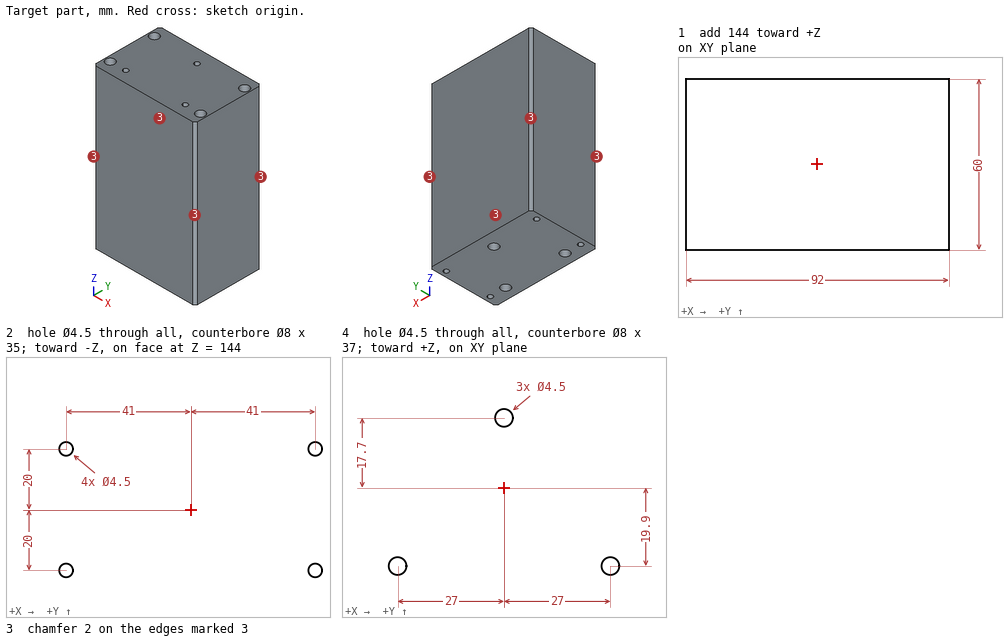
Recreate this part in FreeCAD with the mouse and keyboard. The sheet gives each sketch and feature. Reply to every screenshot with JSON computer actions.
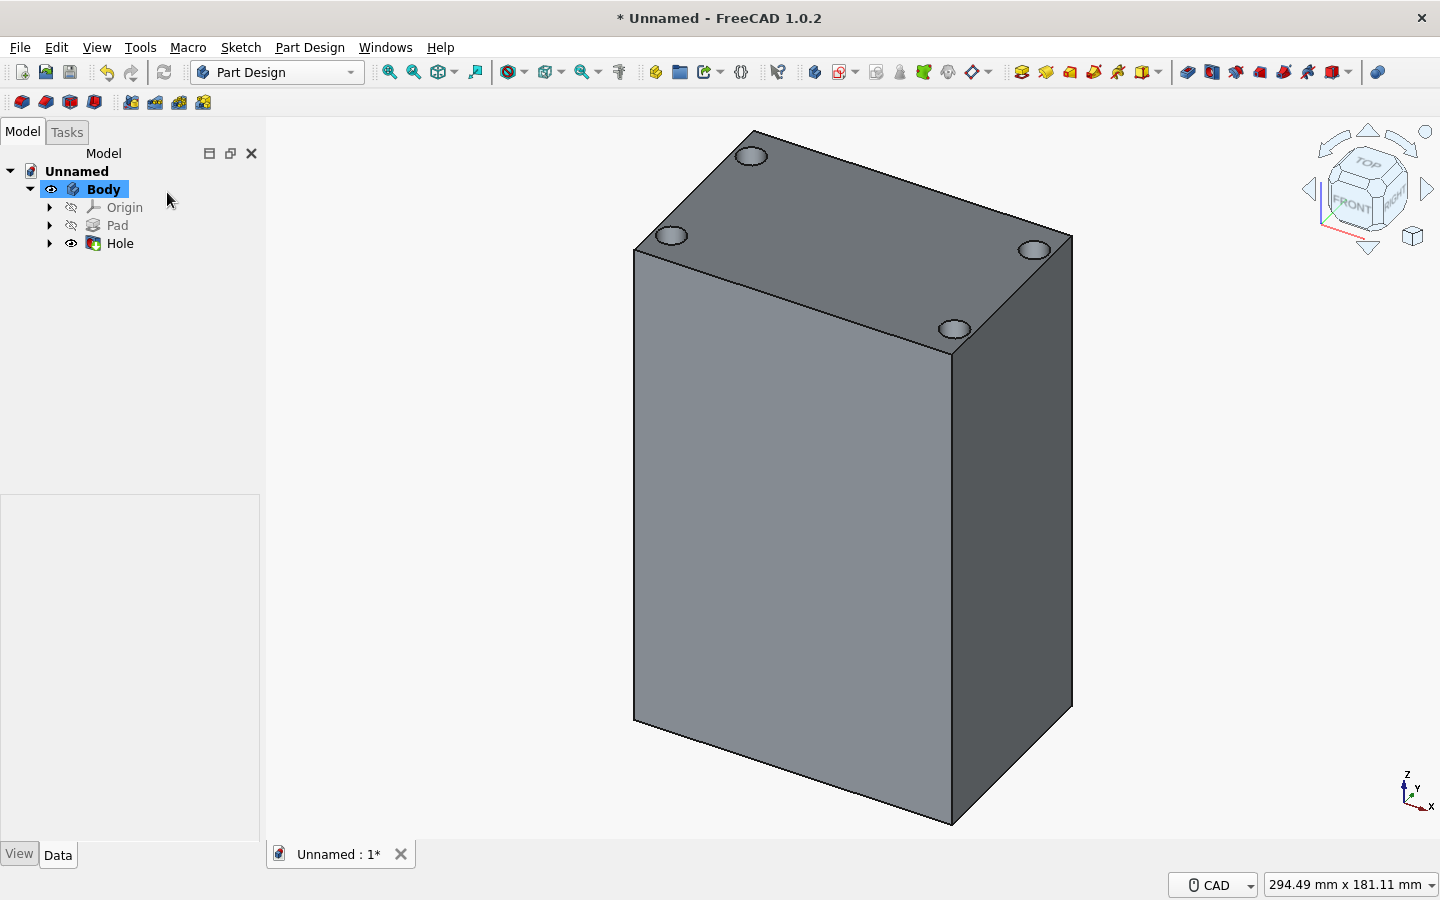
{"action": "left_click", "coordinate": [952, 589]}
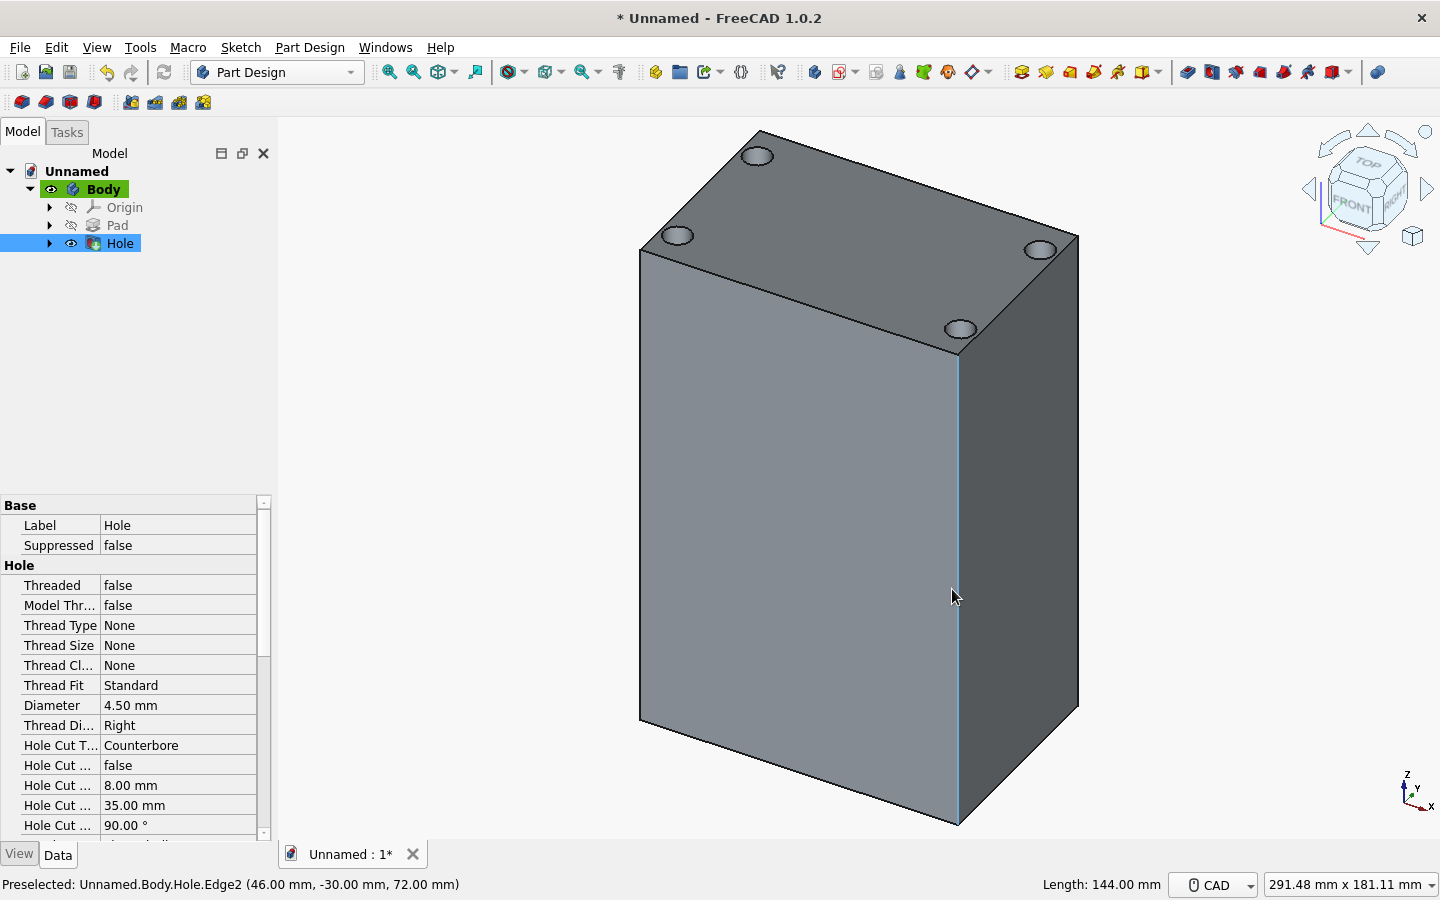
{"action": "key", "text": "0"}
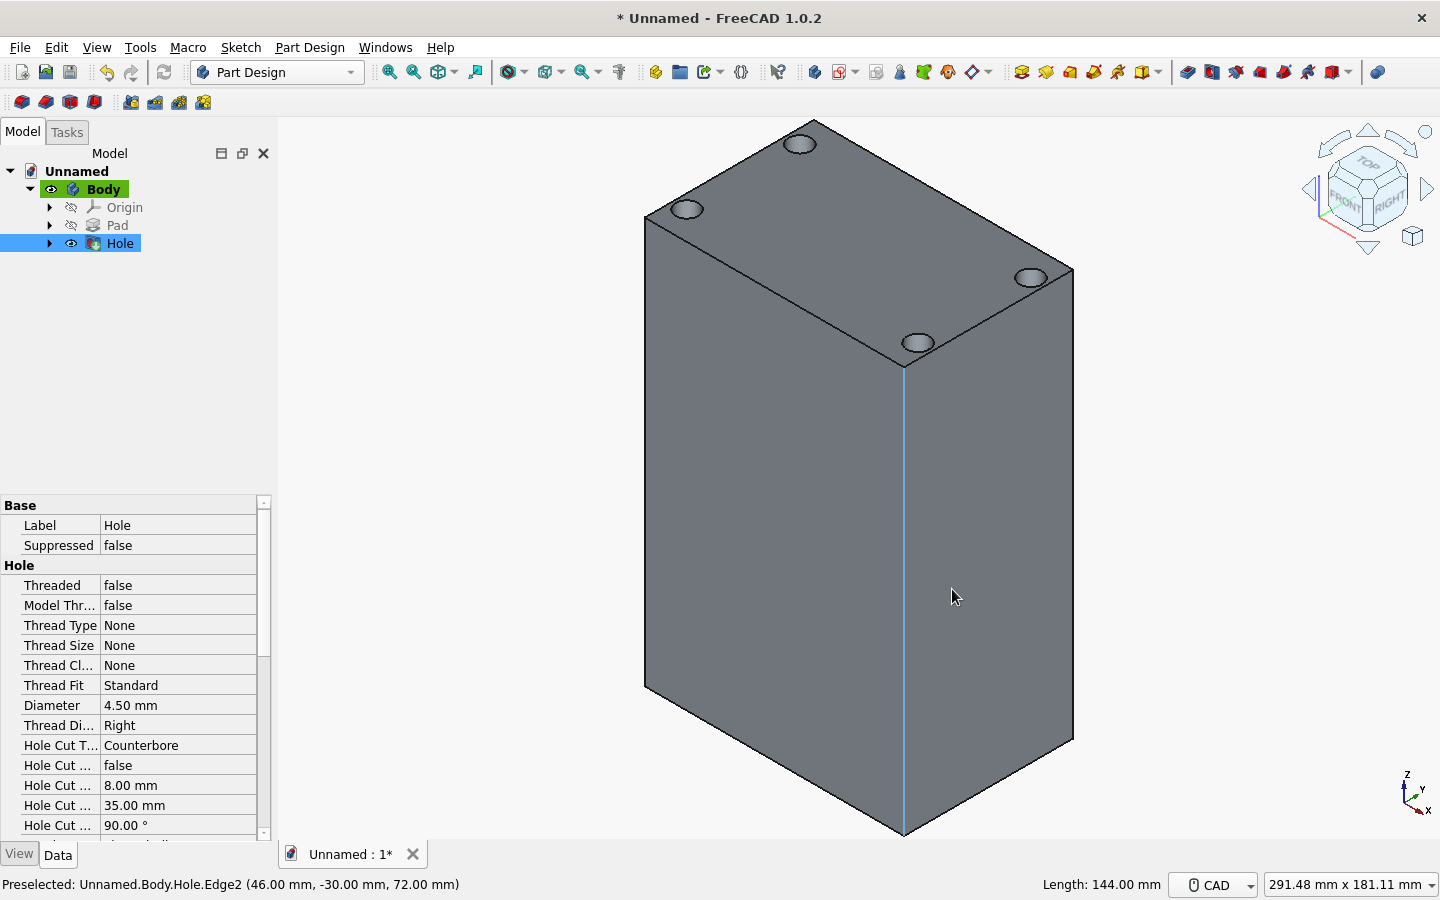
{"action": "key", "text": "2"}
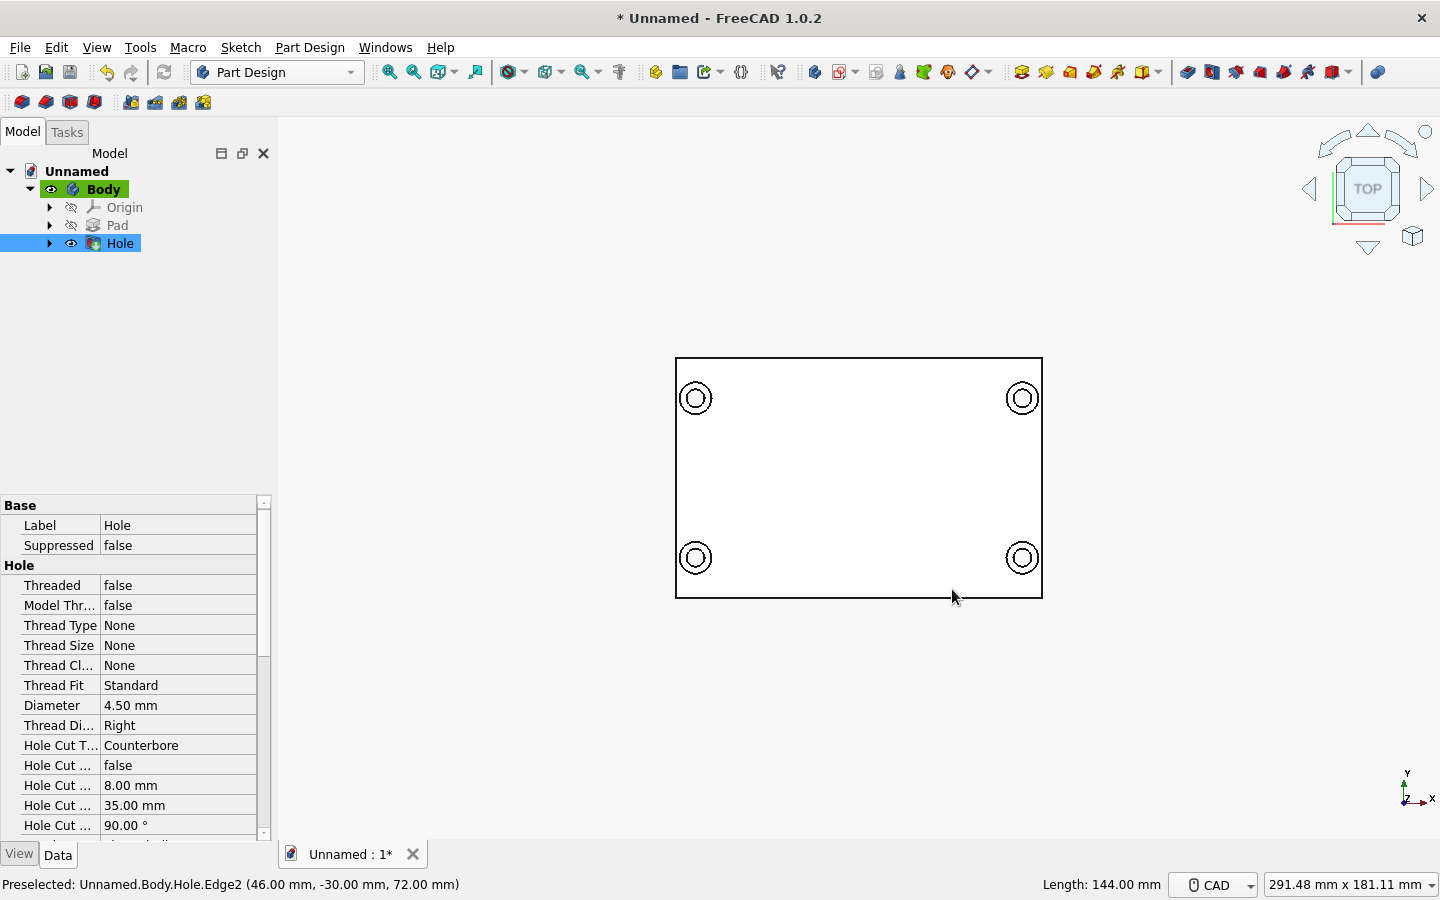
{"action": "left_click", "coordinate": [390, 72]}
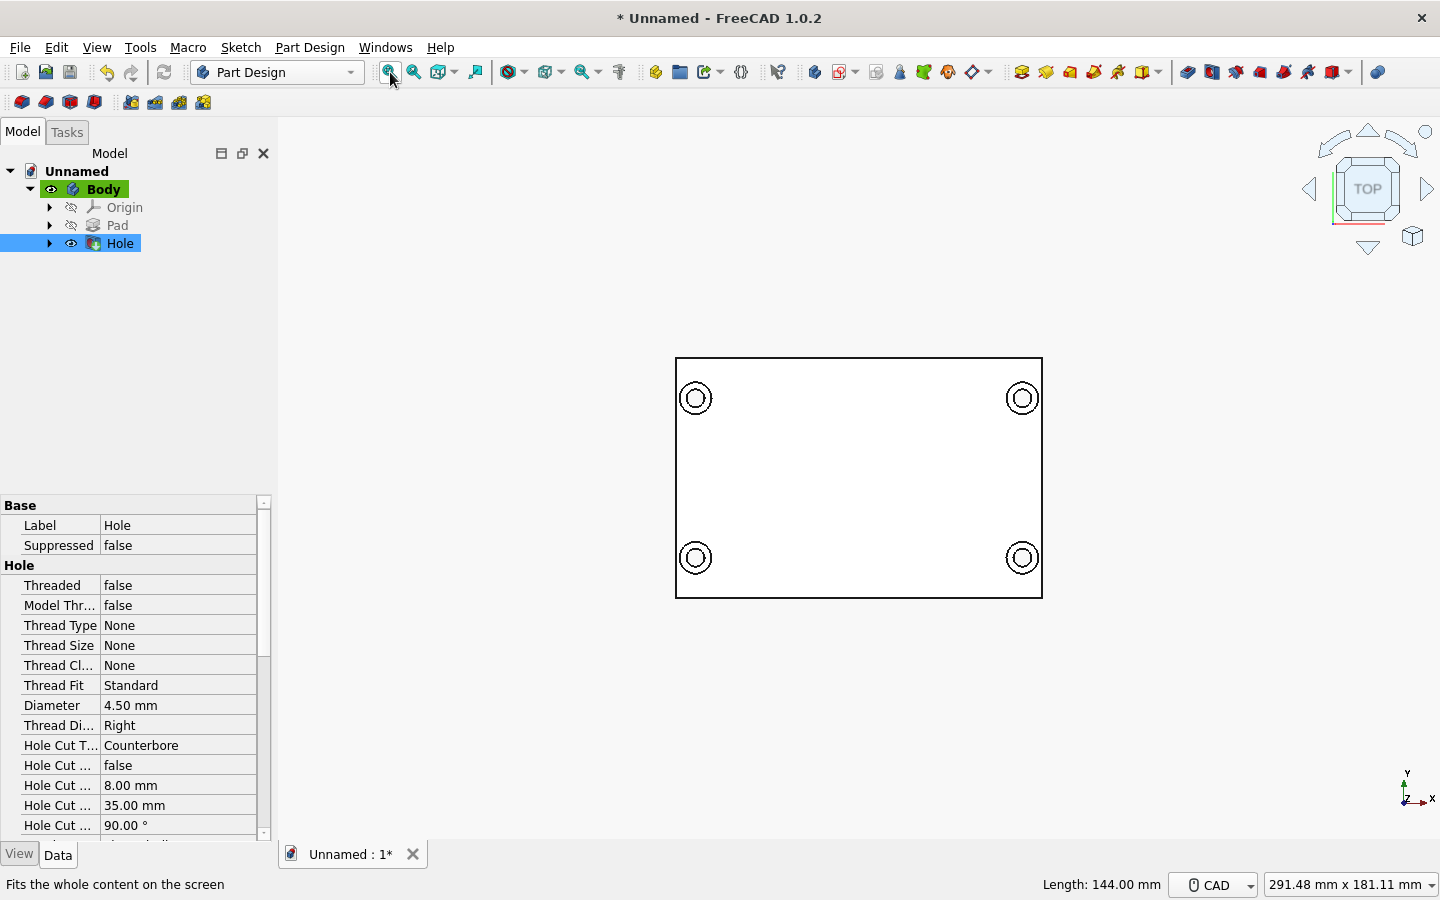
{"action": "key", "text": "1"}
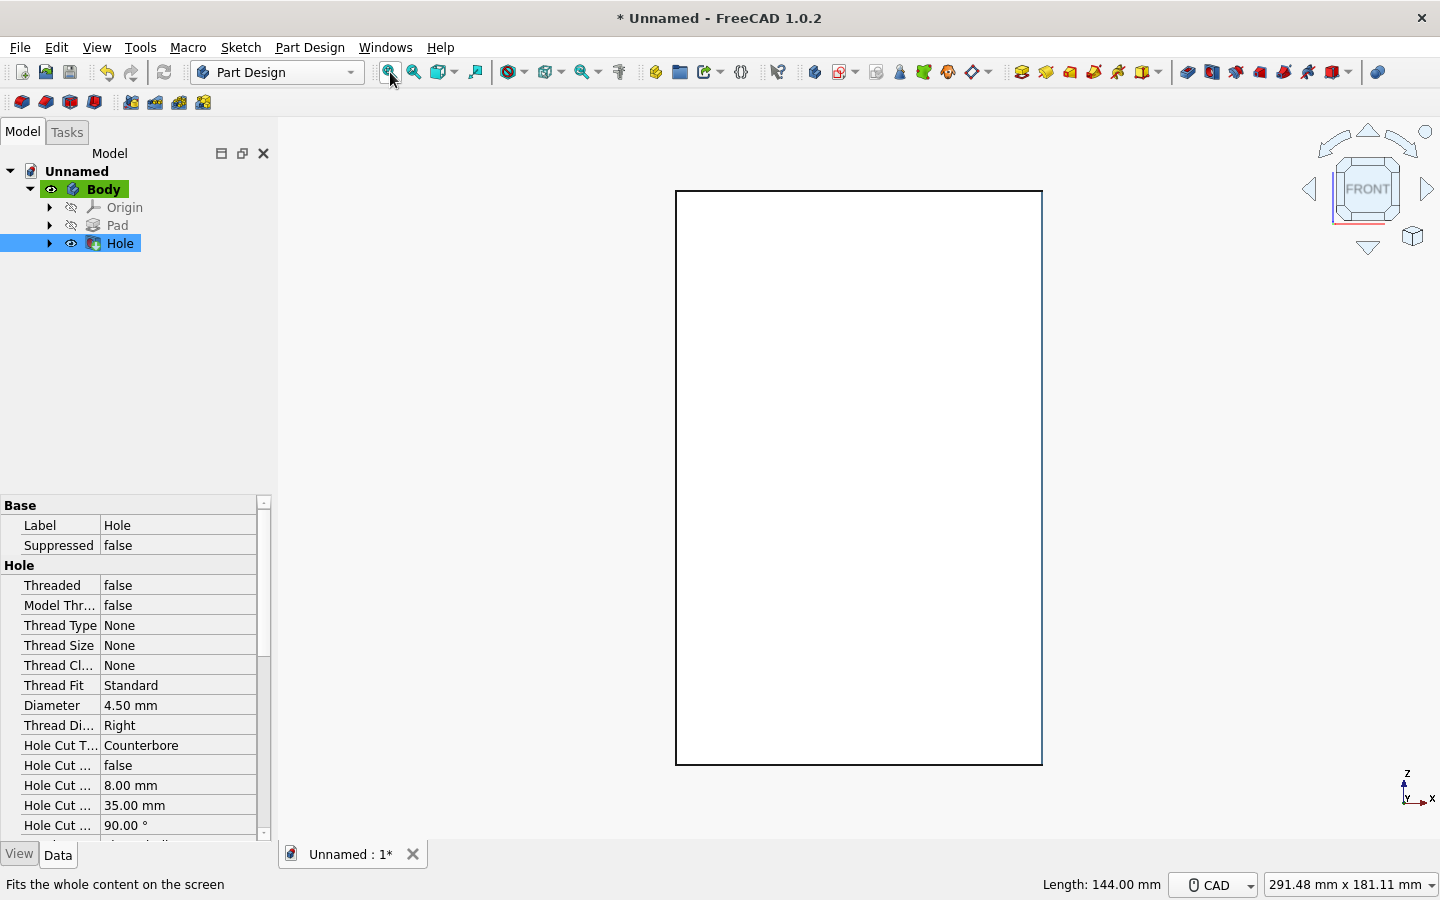
{"action": "left_click", "coordinate": [676, 477], "text": "ctrl"}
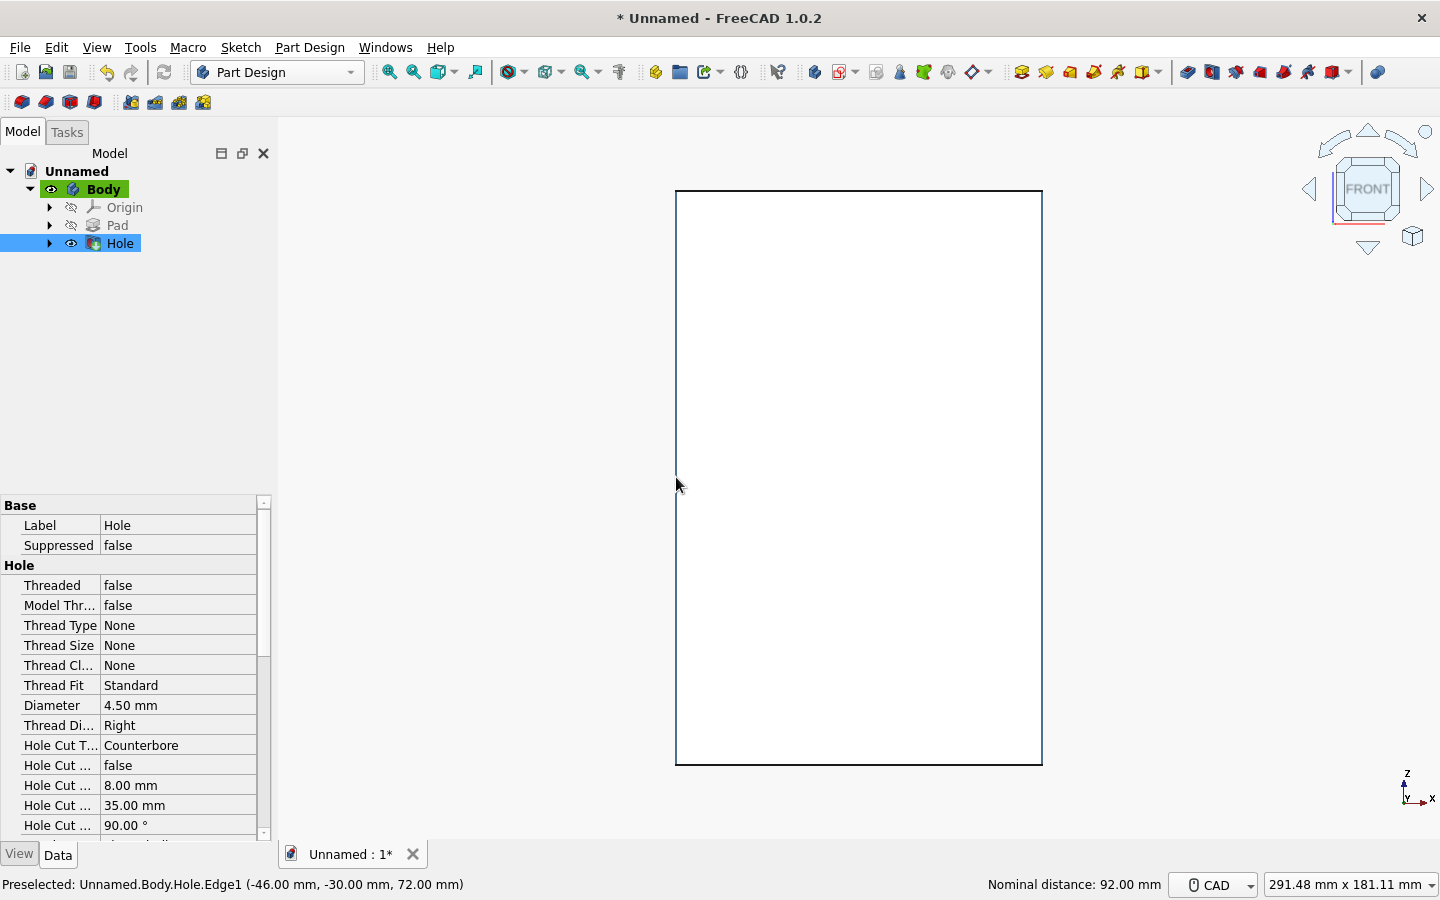
{"action": "key", "text": "3"}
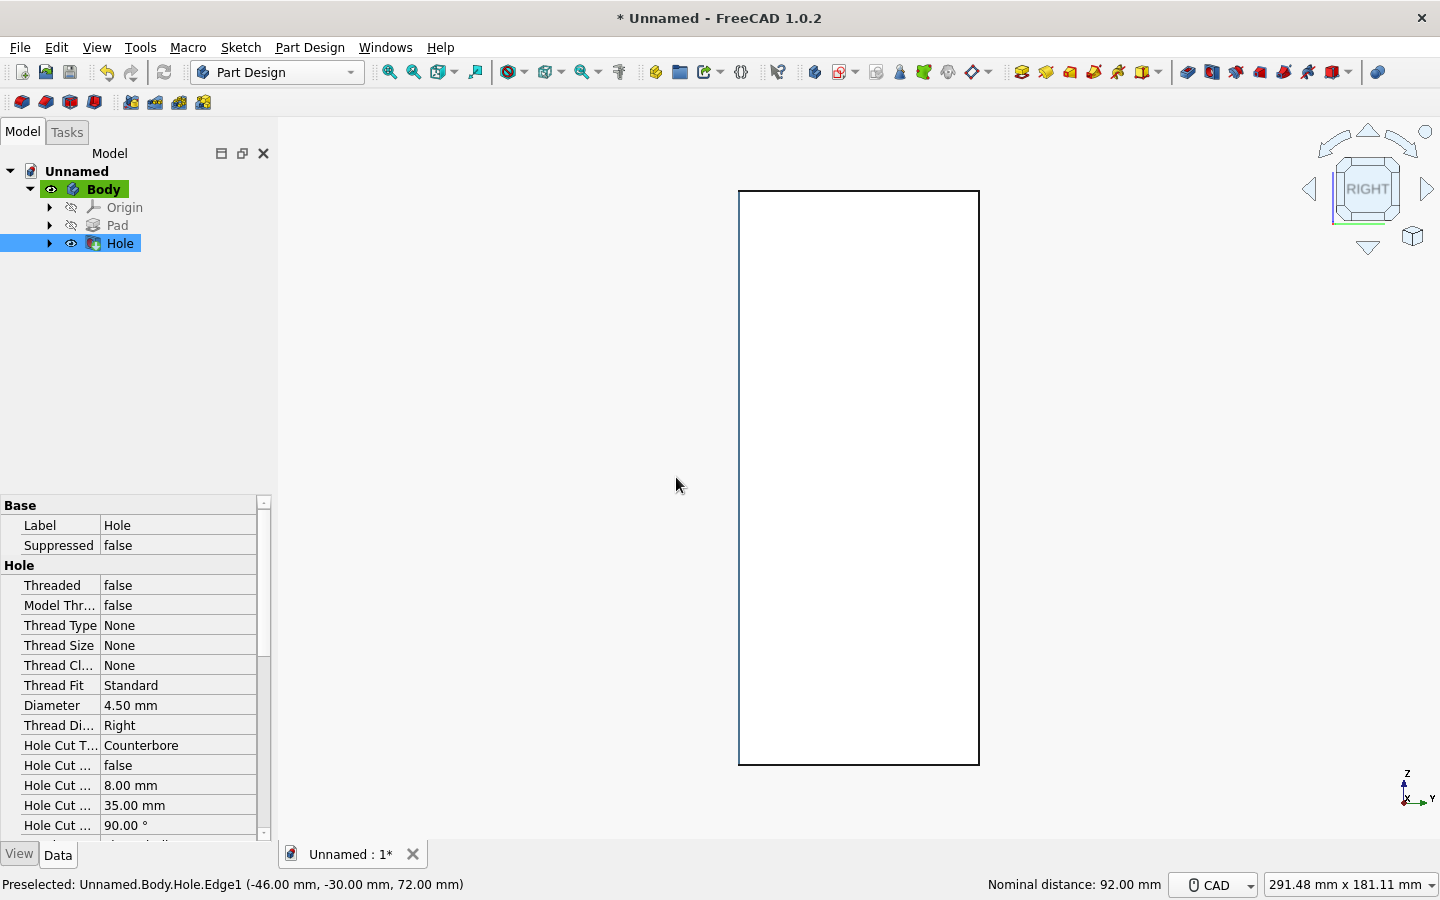
{"action": "left_click", "coordinate": [979, 477], "text": "ctrl"}